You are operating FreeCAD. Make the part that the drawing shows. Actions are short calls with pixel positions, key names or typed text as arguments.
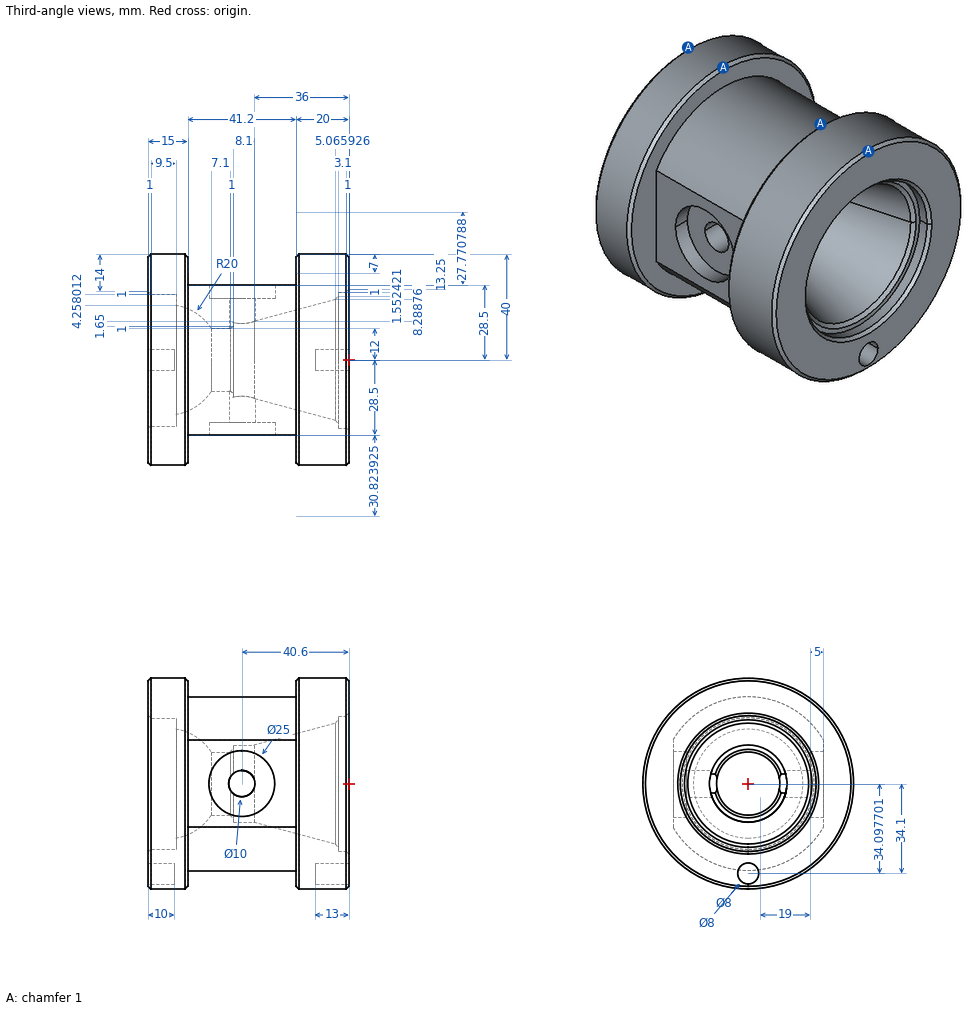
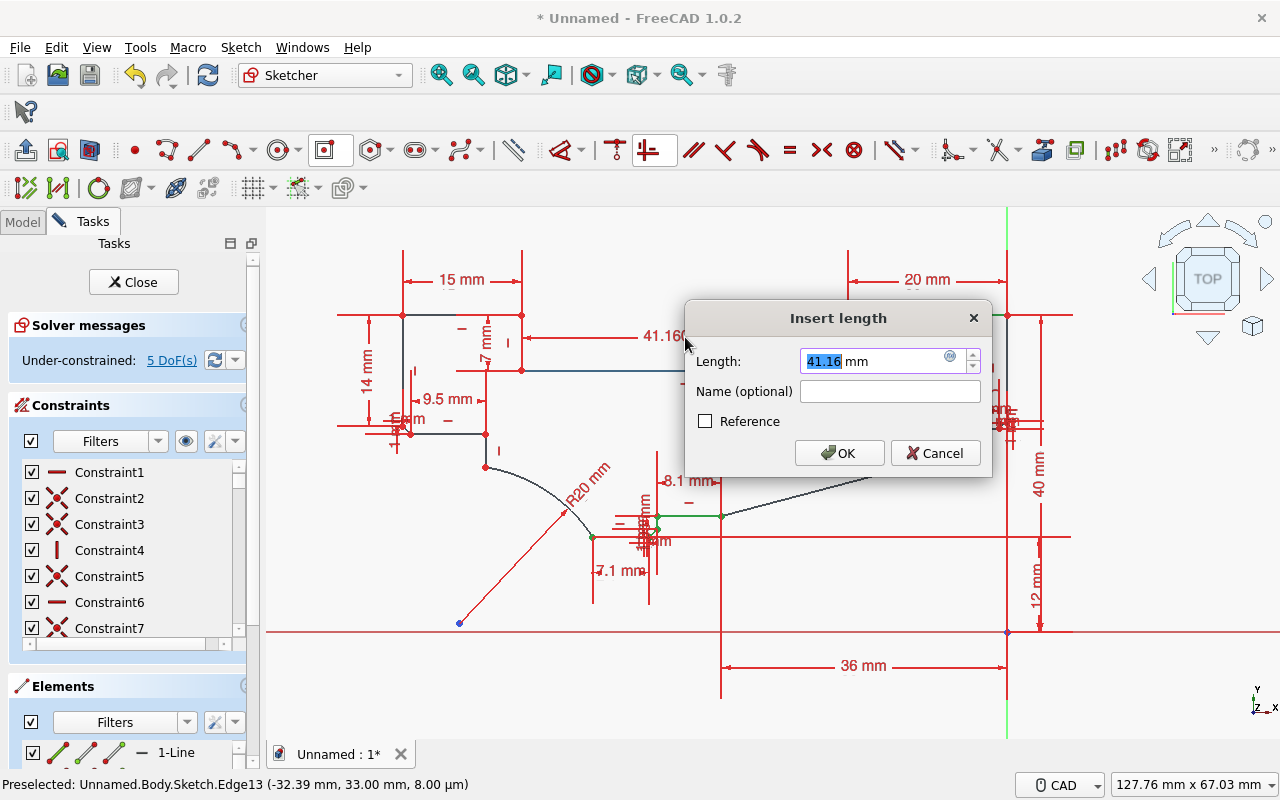
text(41.2)
key(Return)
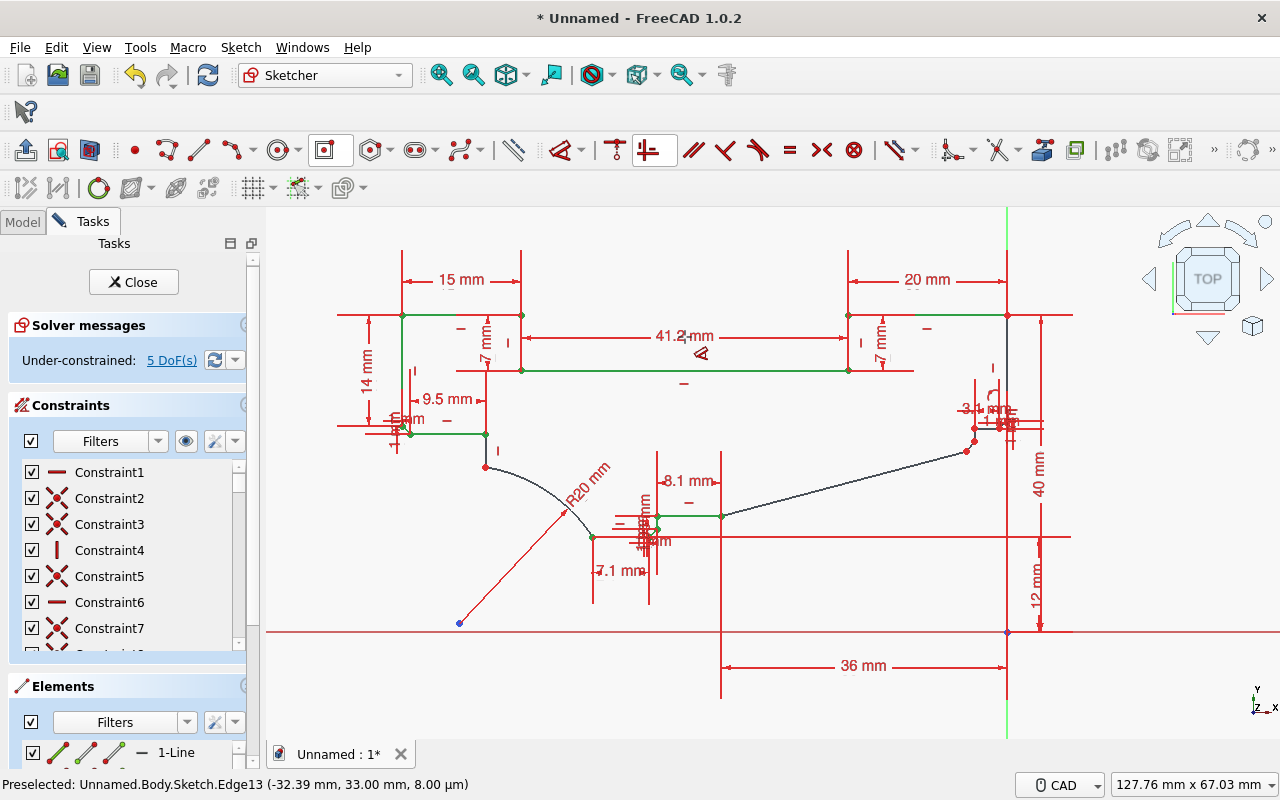
click(1007, 389)
click(1041, 368)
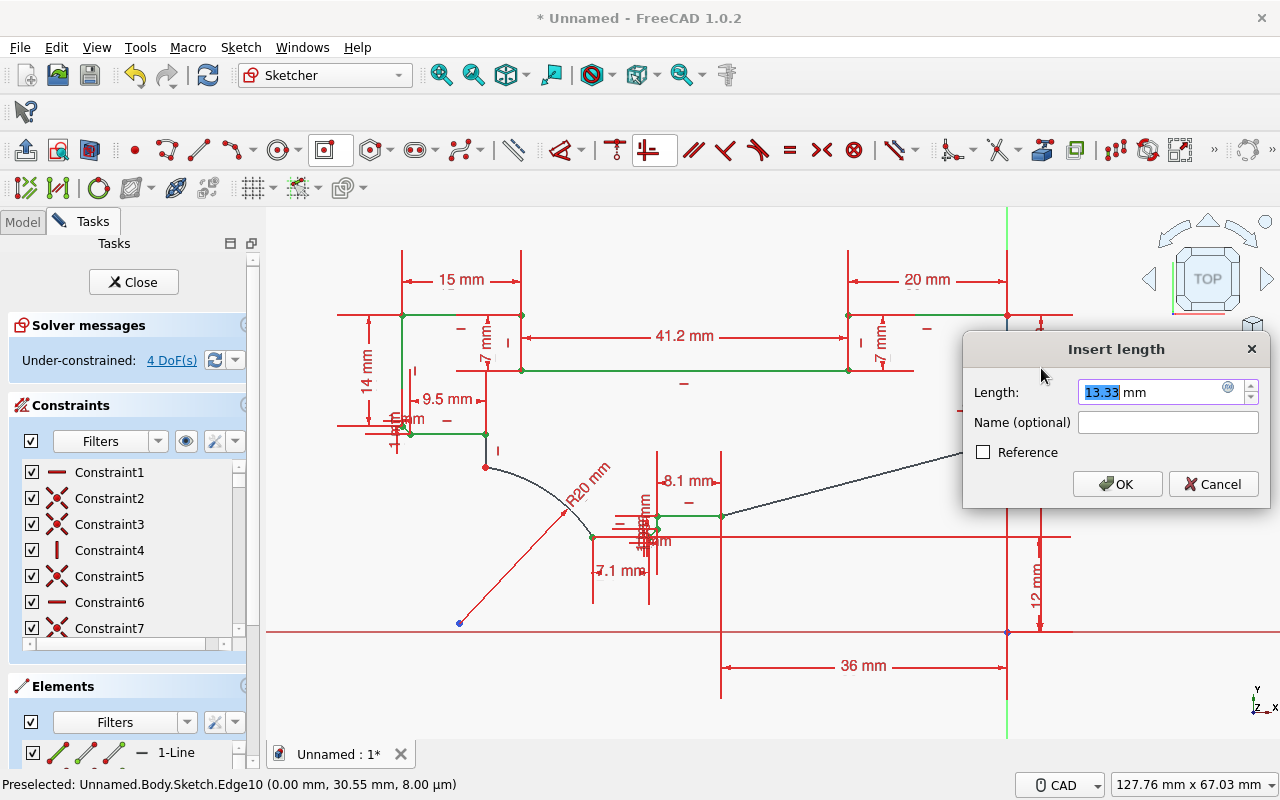
text(13.25)
key(Return)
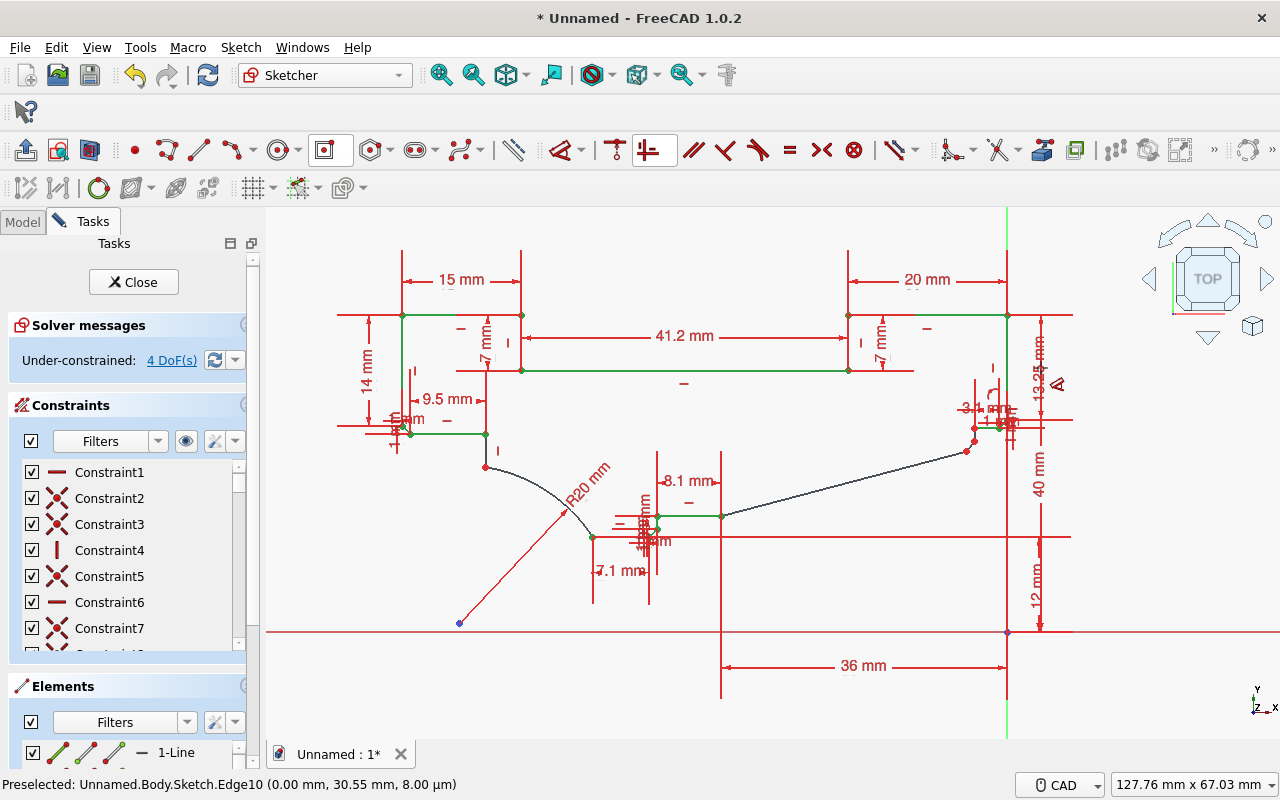
scroll(975, 435, up, 6)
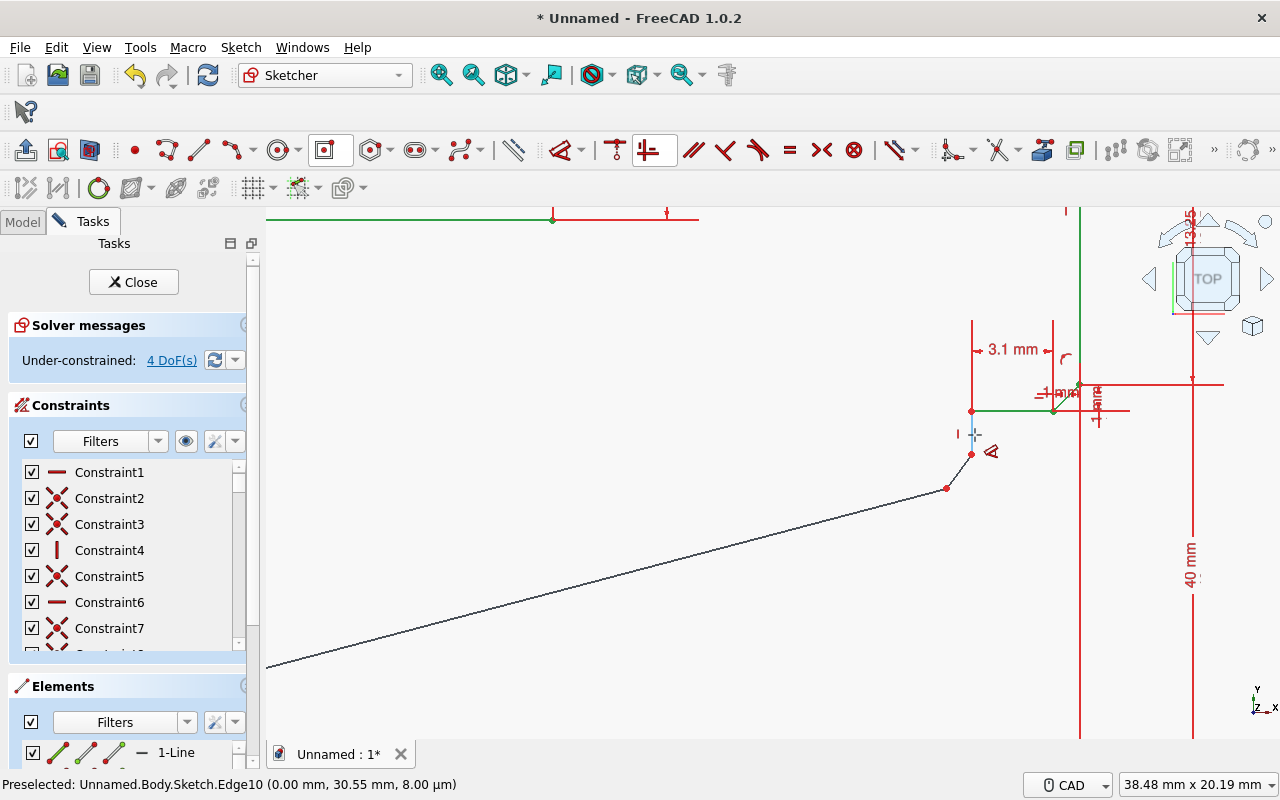
click(972, 433)
click(1006, 433)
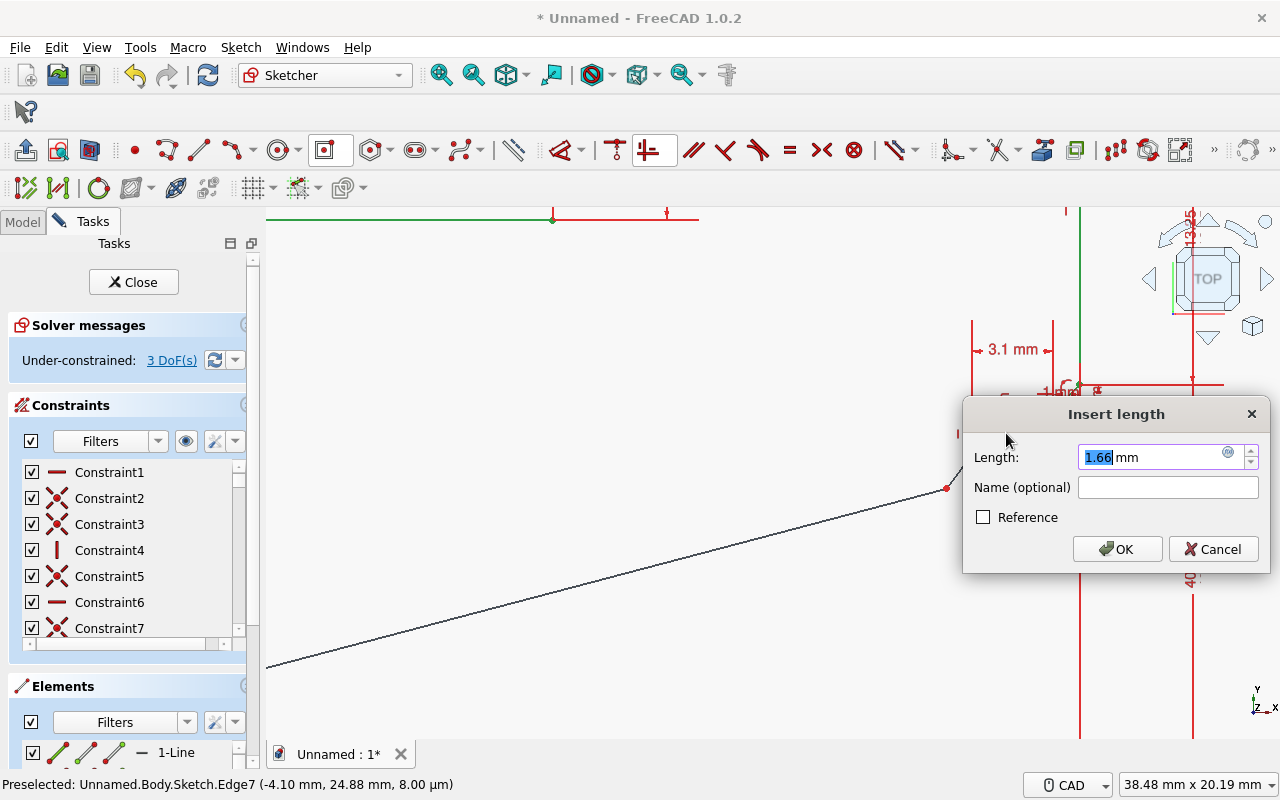
text(1.552421)
key(Return)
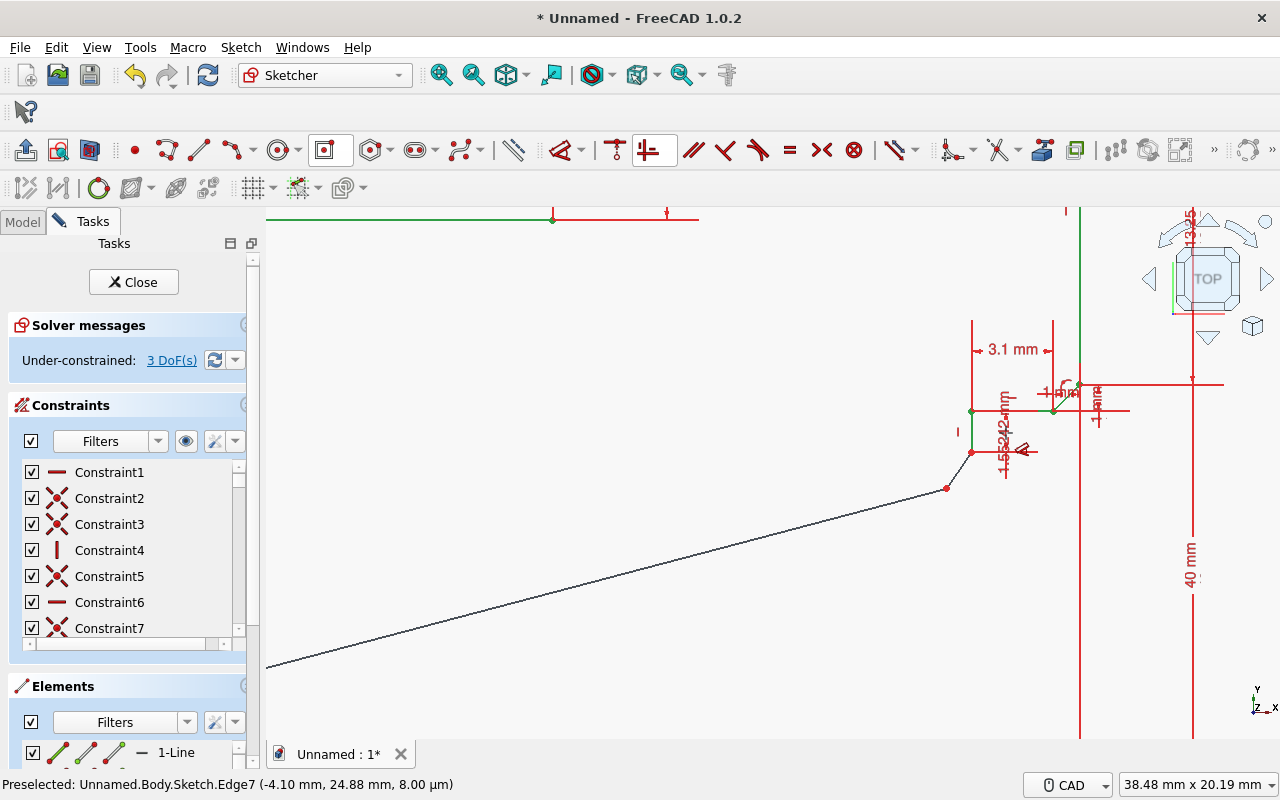
scroll(975, 434, down, 6)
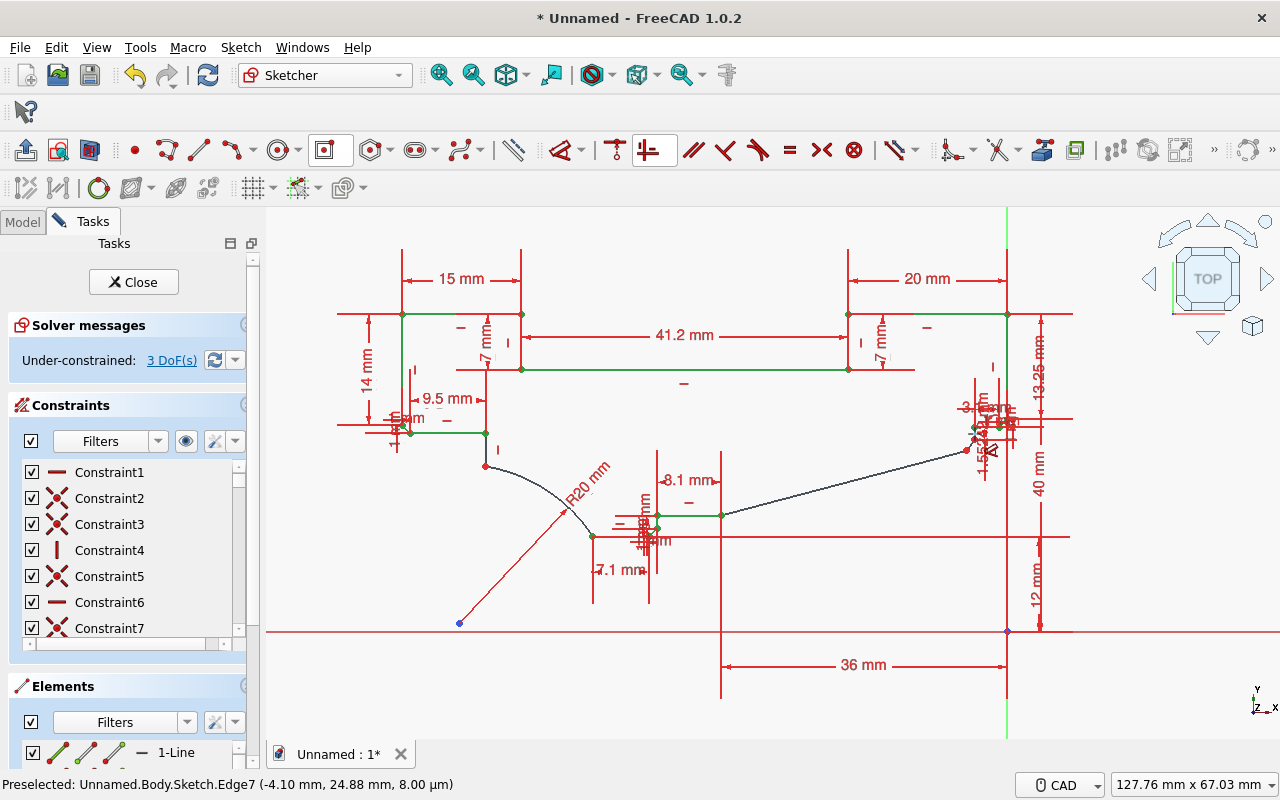
scroll(486, 443, up, 2)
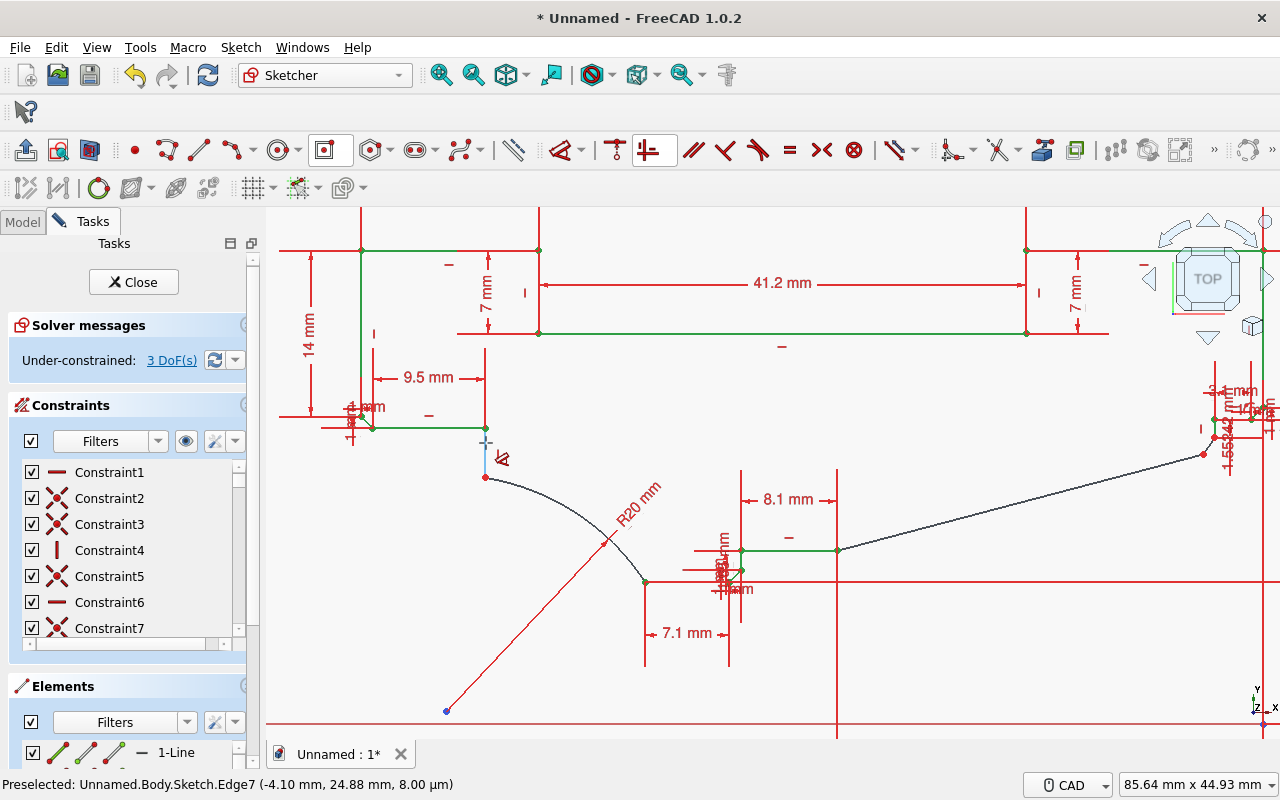
click(485, 443)
click(451, 453)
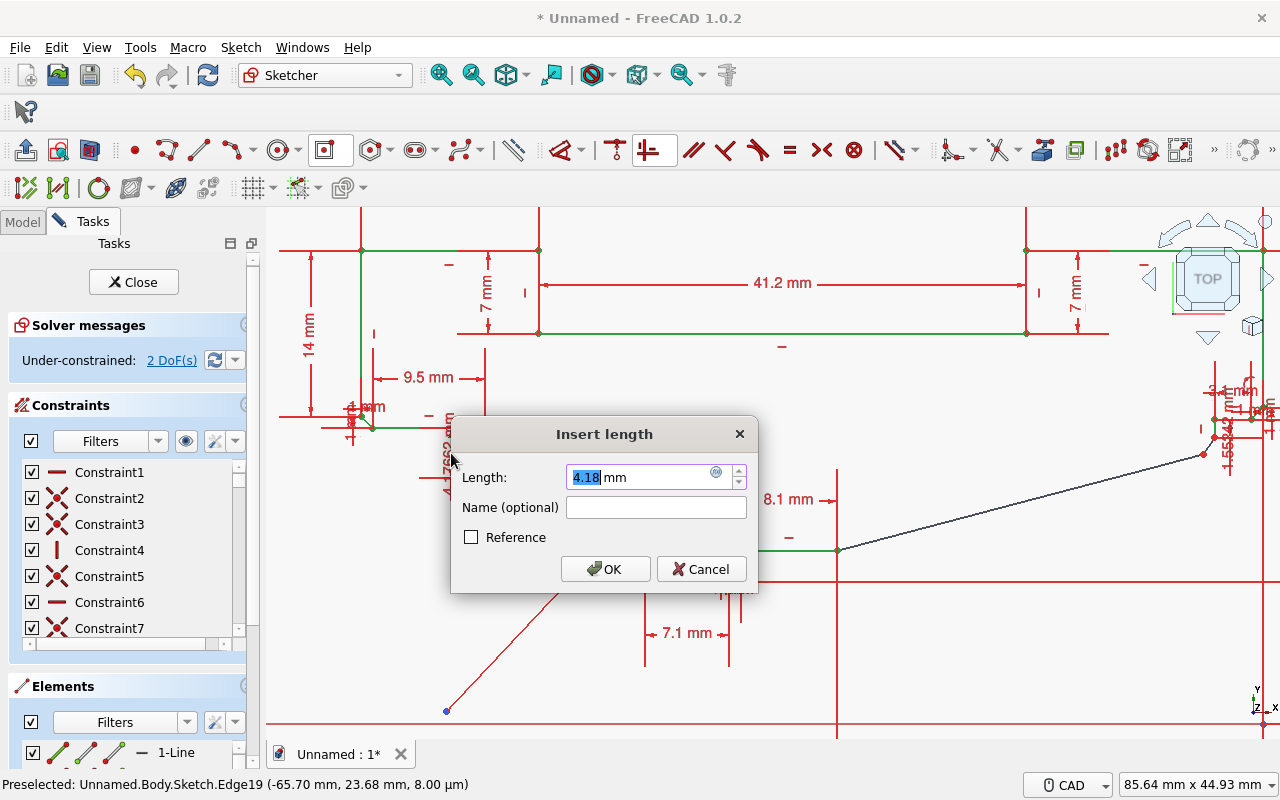
text(4.258012)
key(Return)